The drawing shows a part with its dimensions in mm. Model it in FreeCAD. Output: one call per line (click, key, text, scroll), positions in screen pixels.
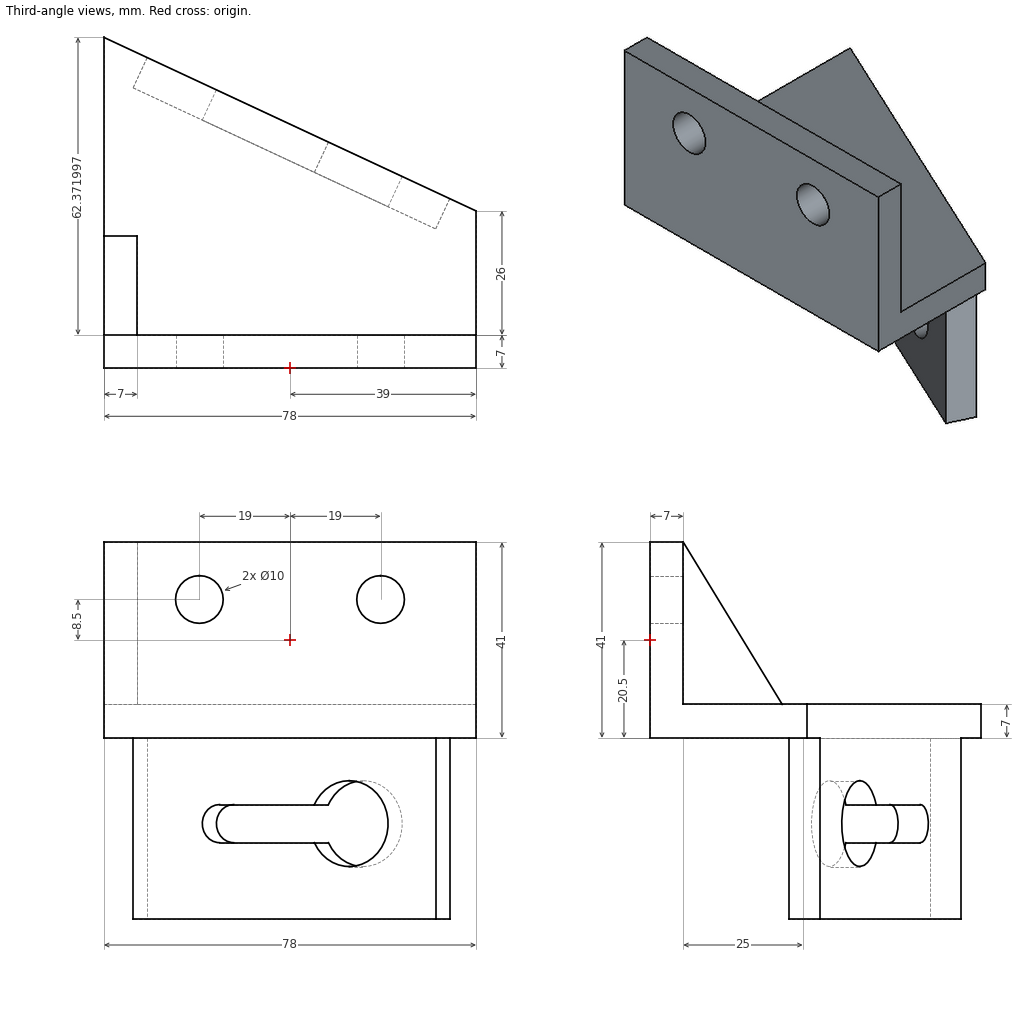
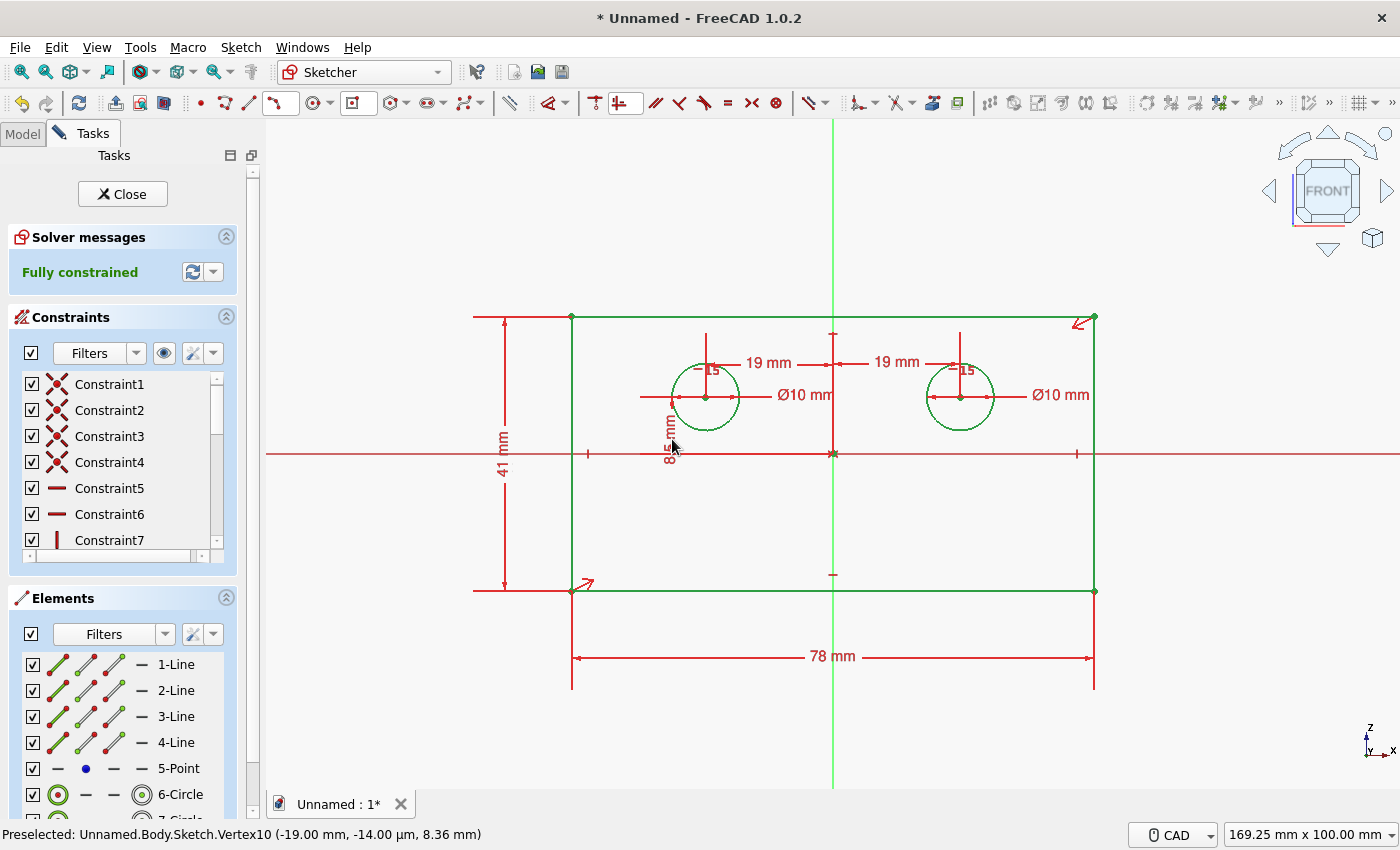
click(123, 194)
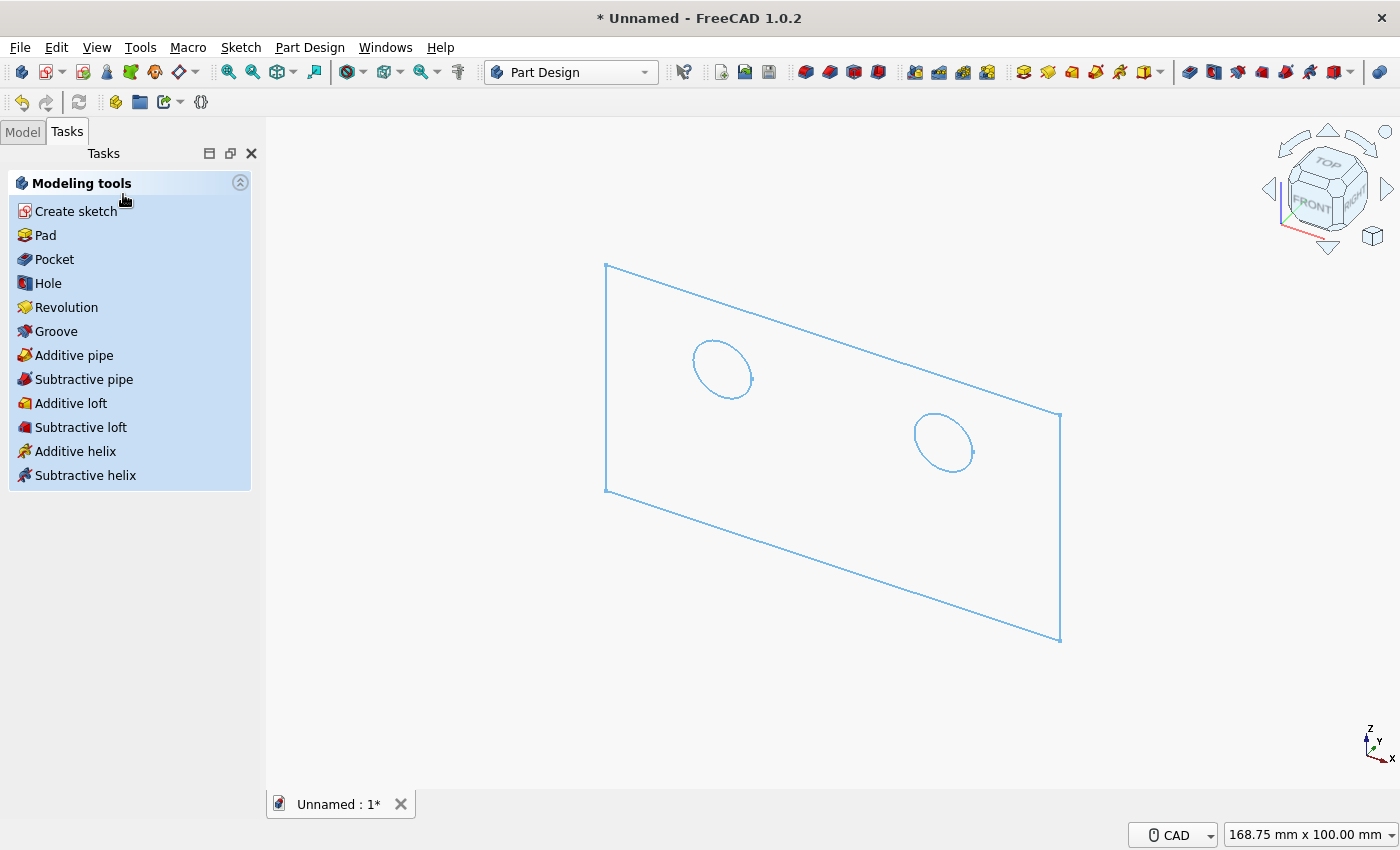
click(1024, 72)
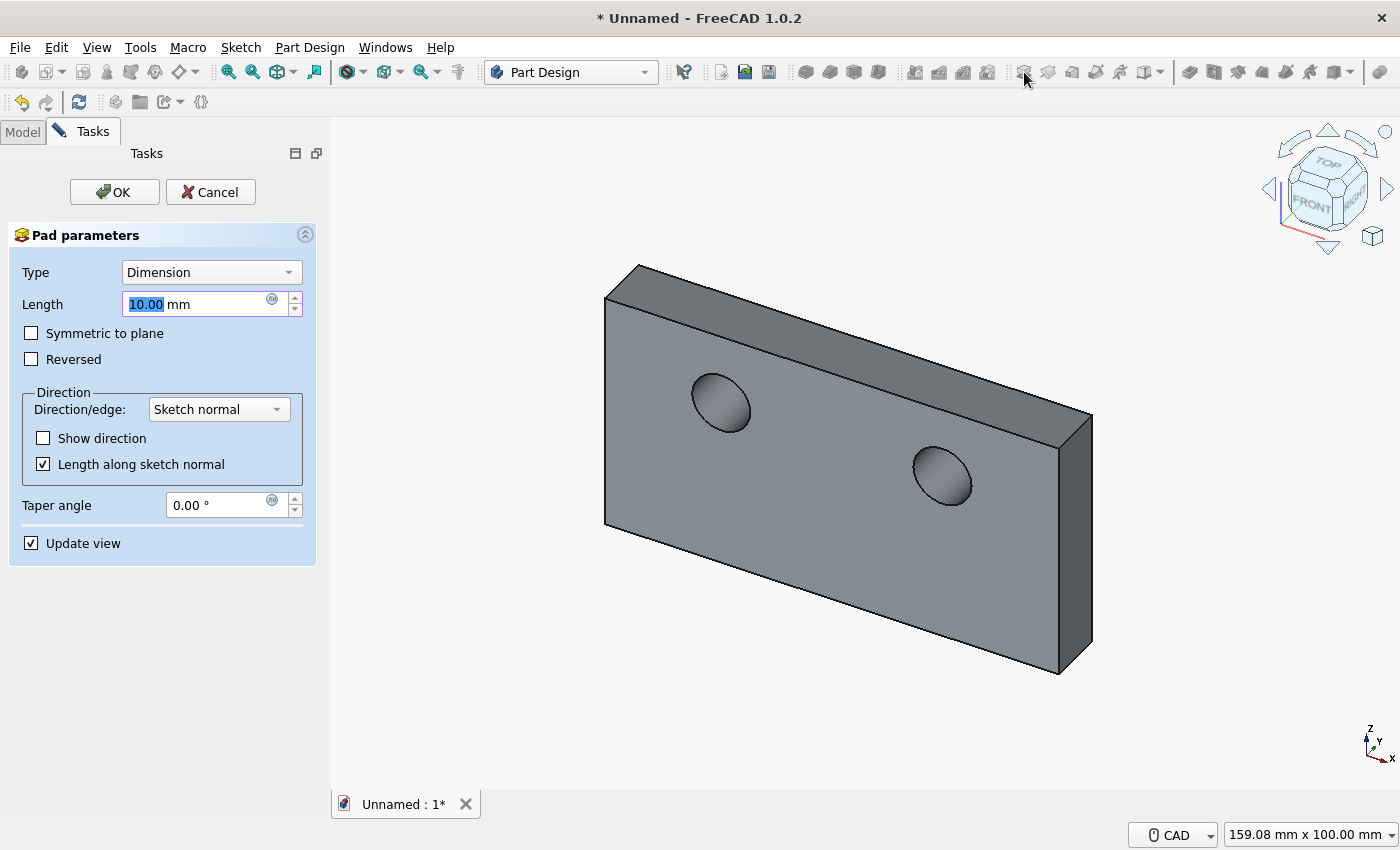
text(7)
key(Tab)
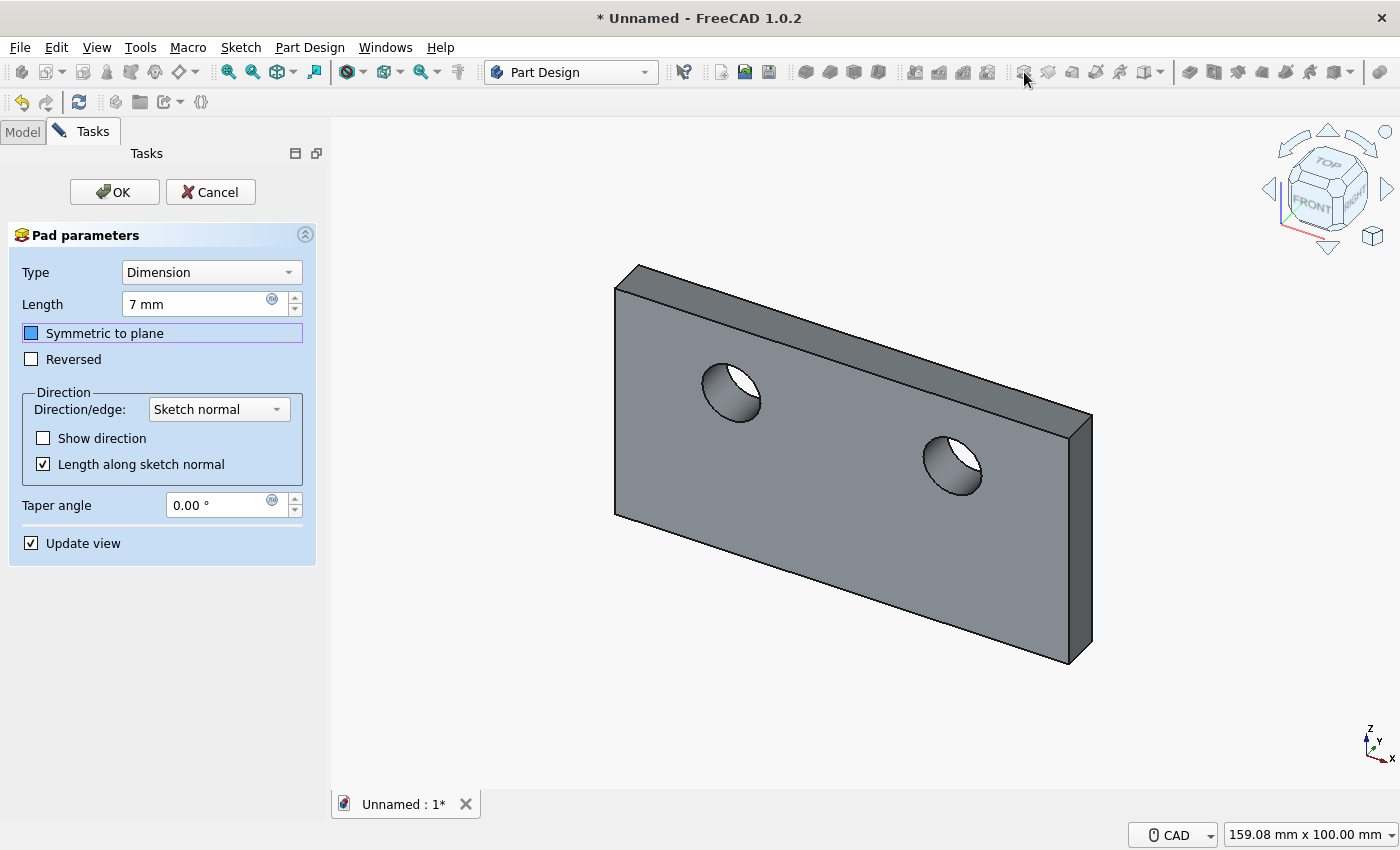
click(30, 359)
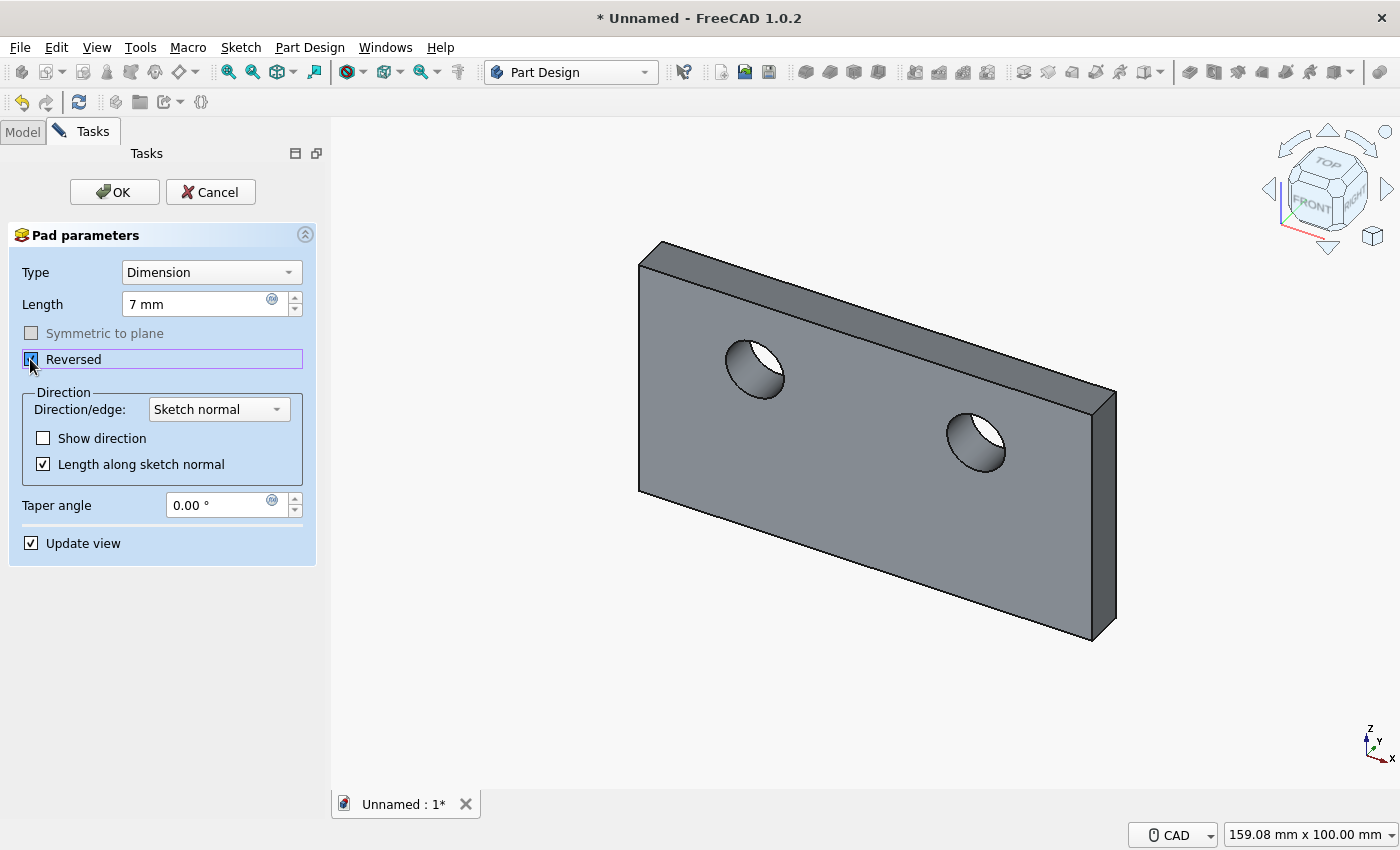
click(115, 192)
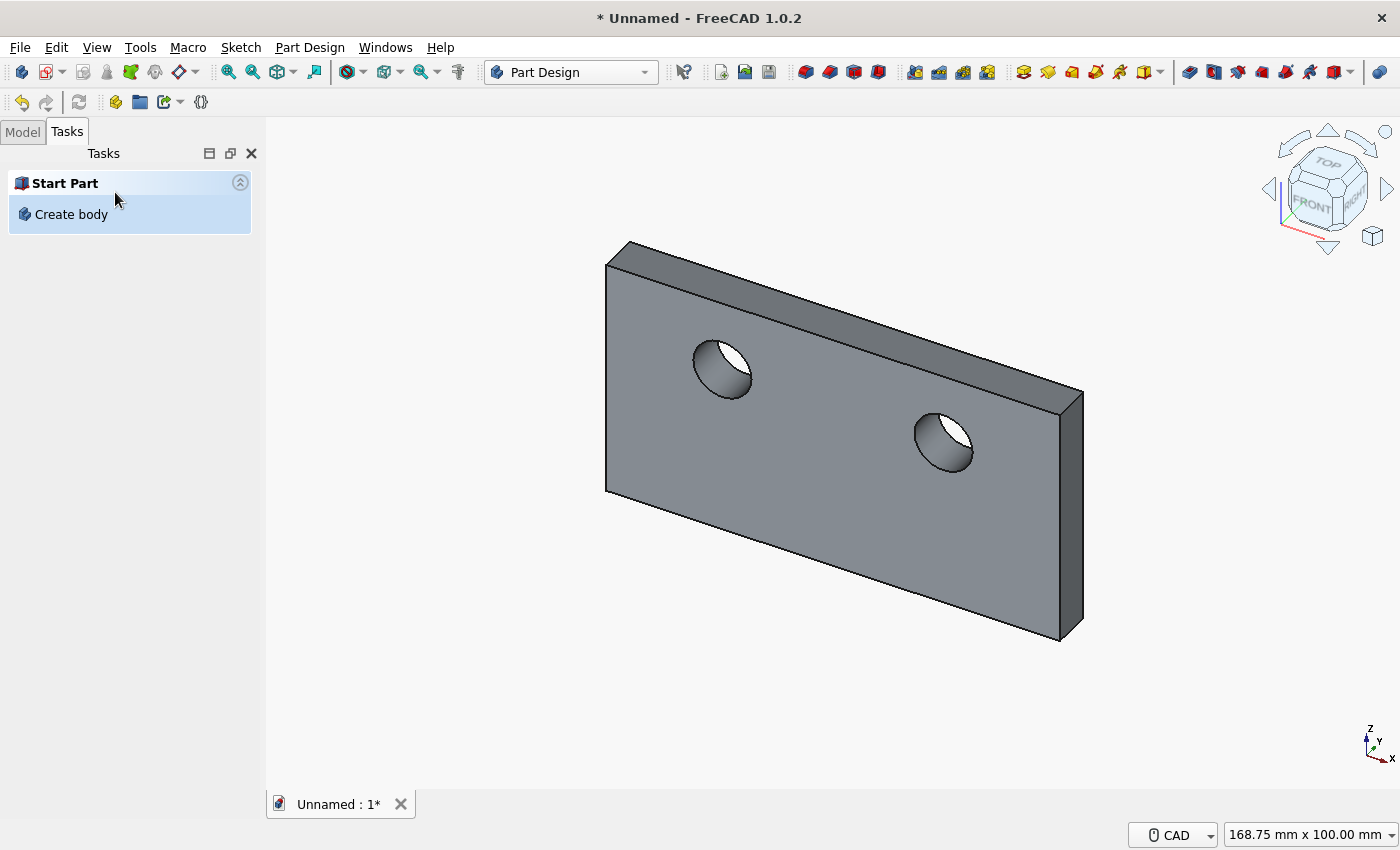
key(6)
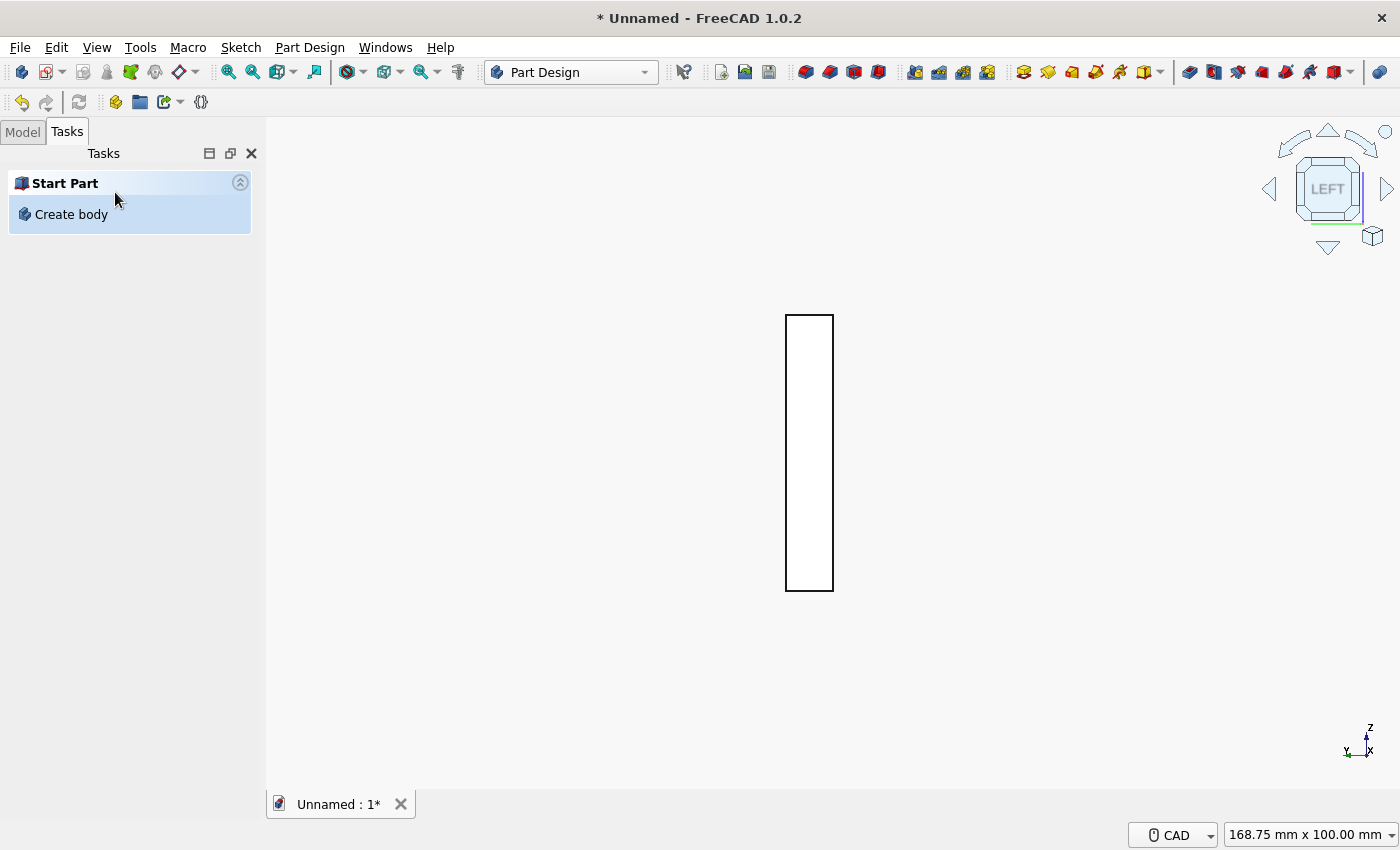
click(230, 72)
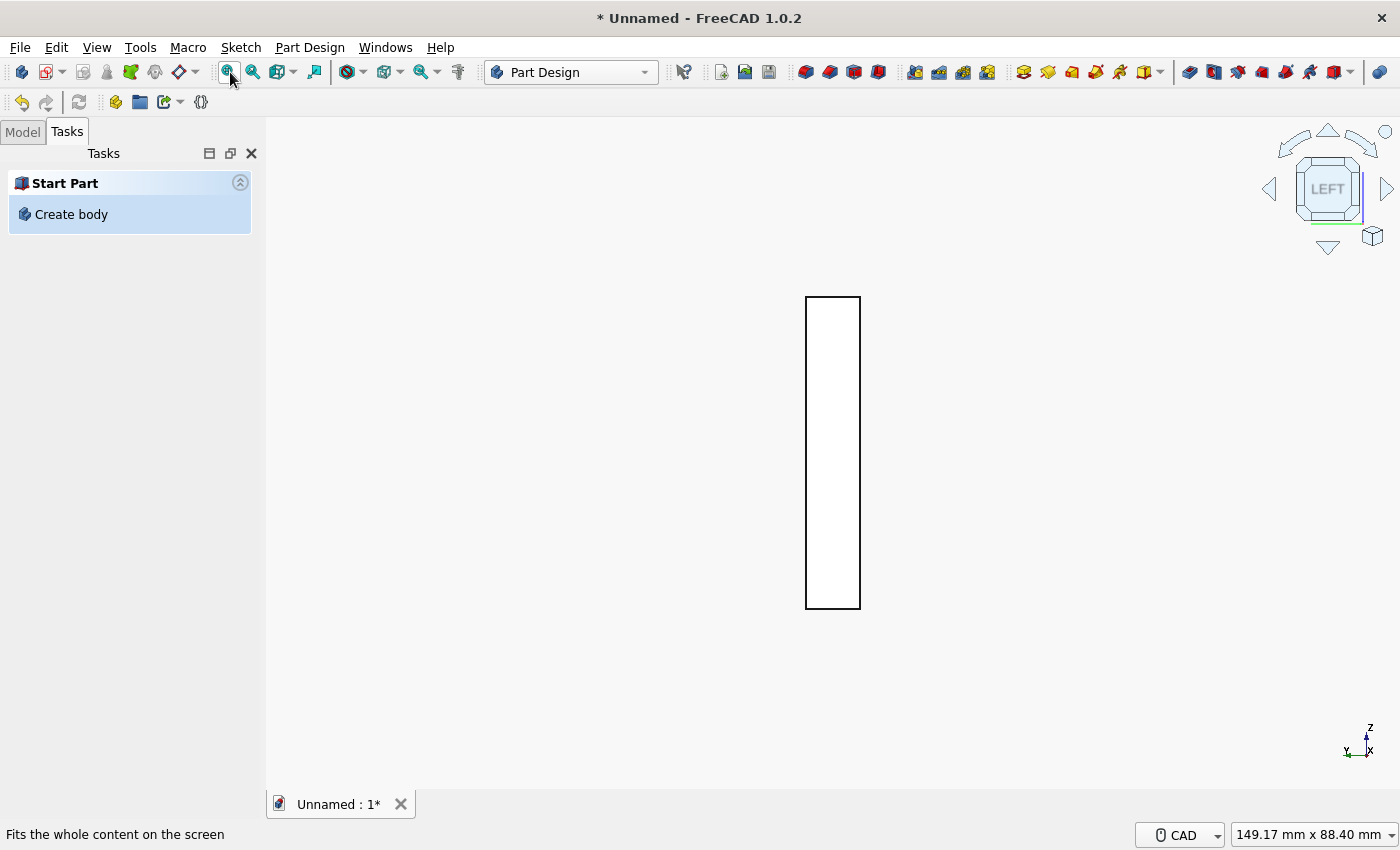
click(833, 363)